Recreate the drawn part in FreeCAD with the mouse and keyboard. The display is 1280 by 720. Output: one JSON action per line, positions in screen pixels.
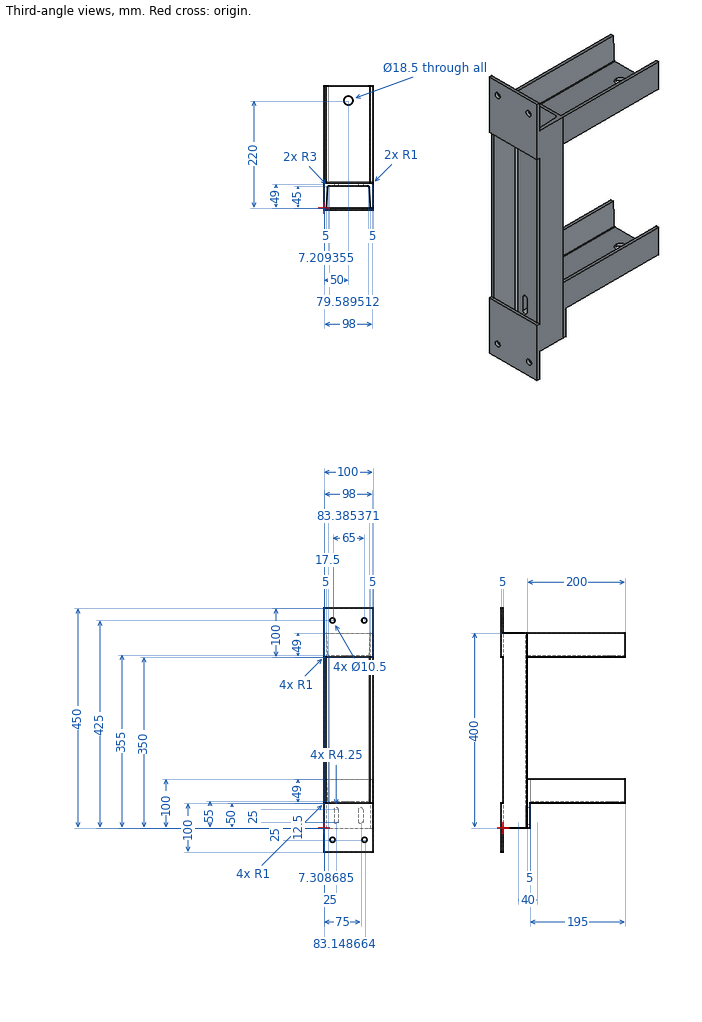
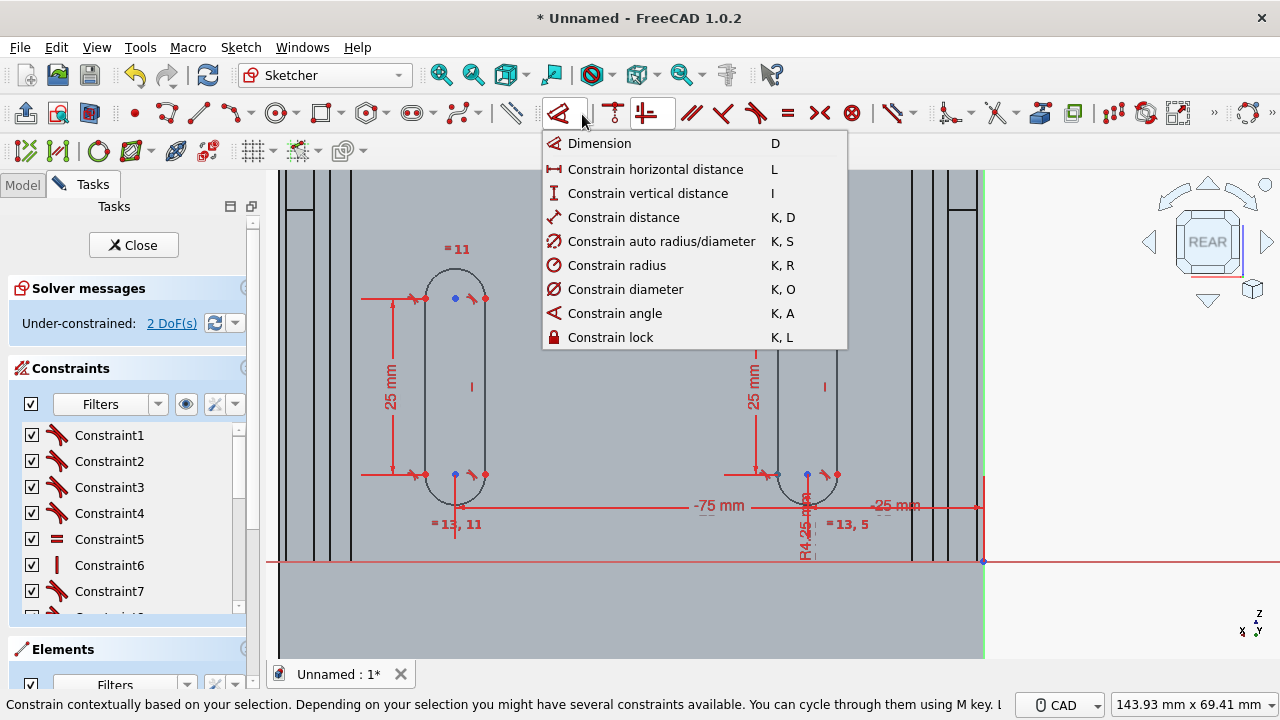
{"action": "left_click", "coordinate": [695, 193]}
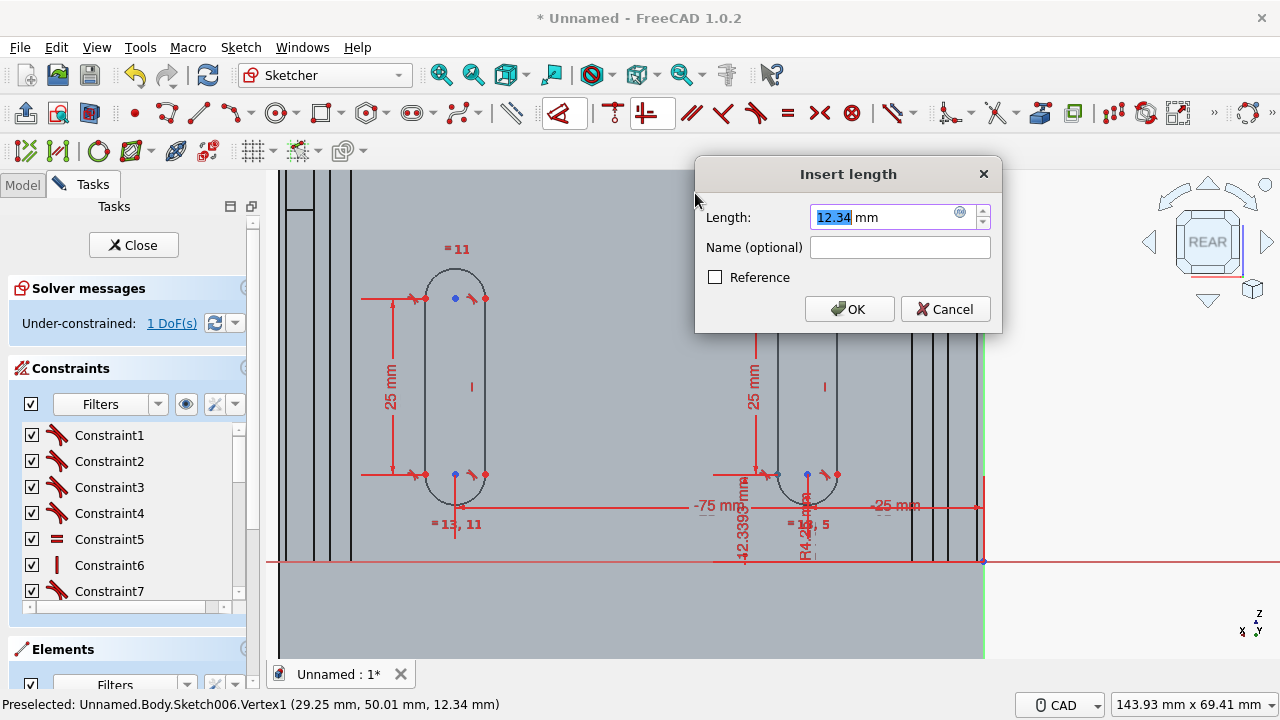
{"action": "type", "text": "12.5"}
{"action": "key", "text": "Return"}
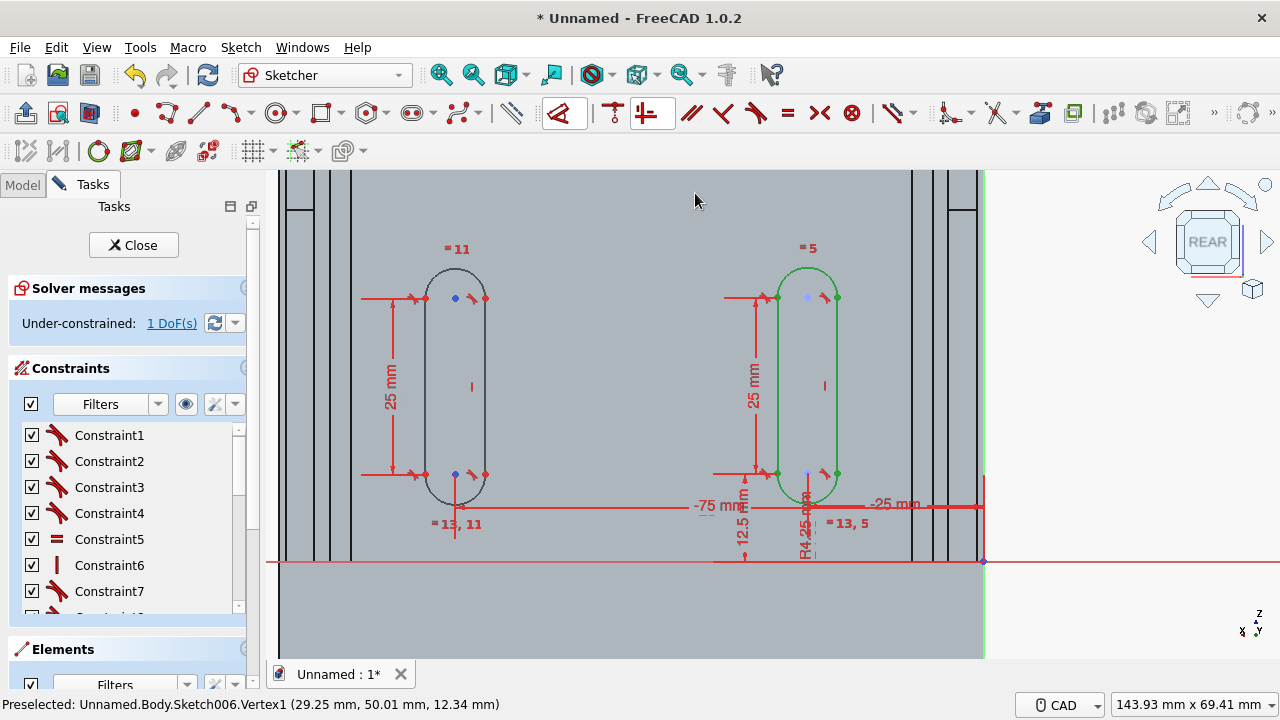
{"action": "left_click", "coordinate": [425, 475]}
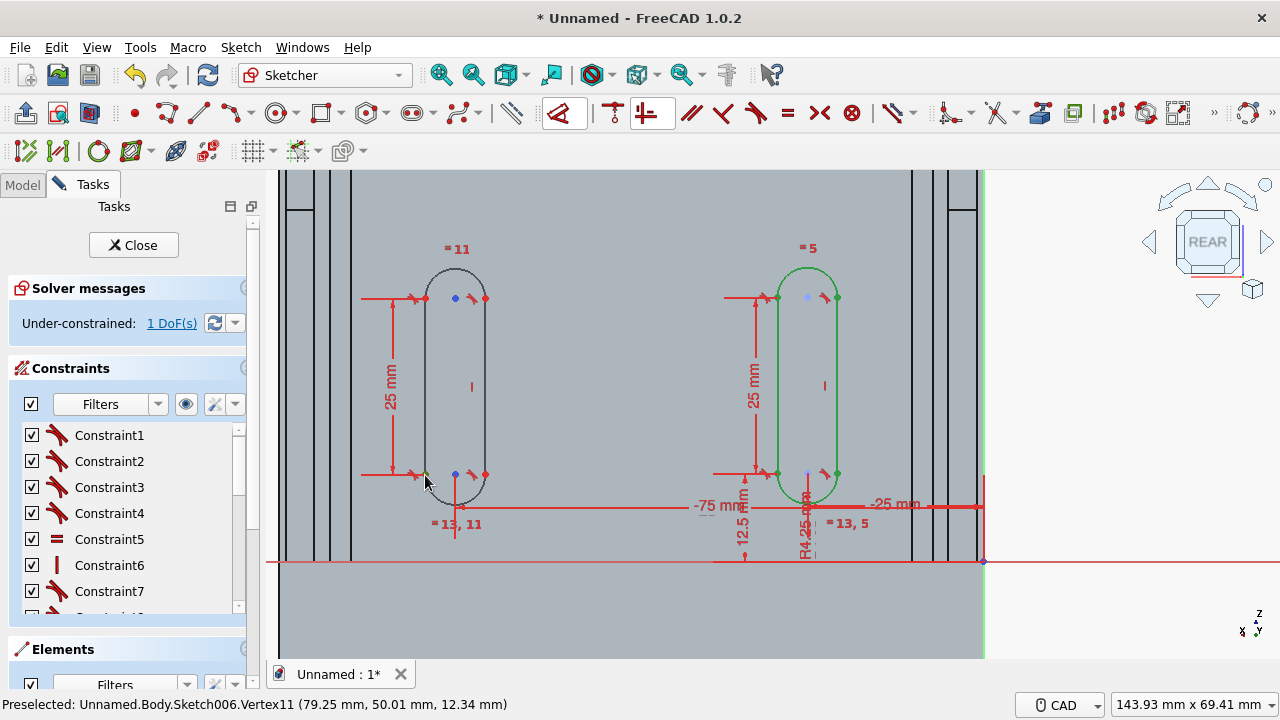
{"action": "key", "text": "i"}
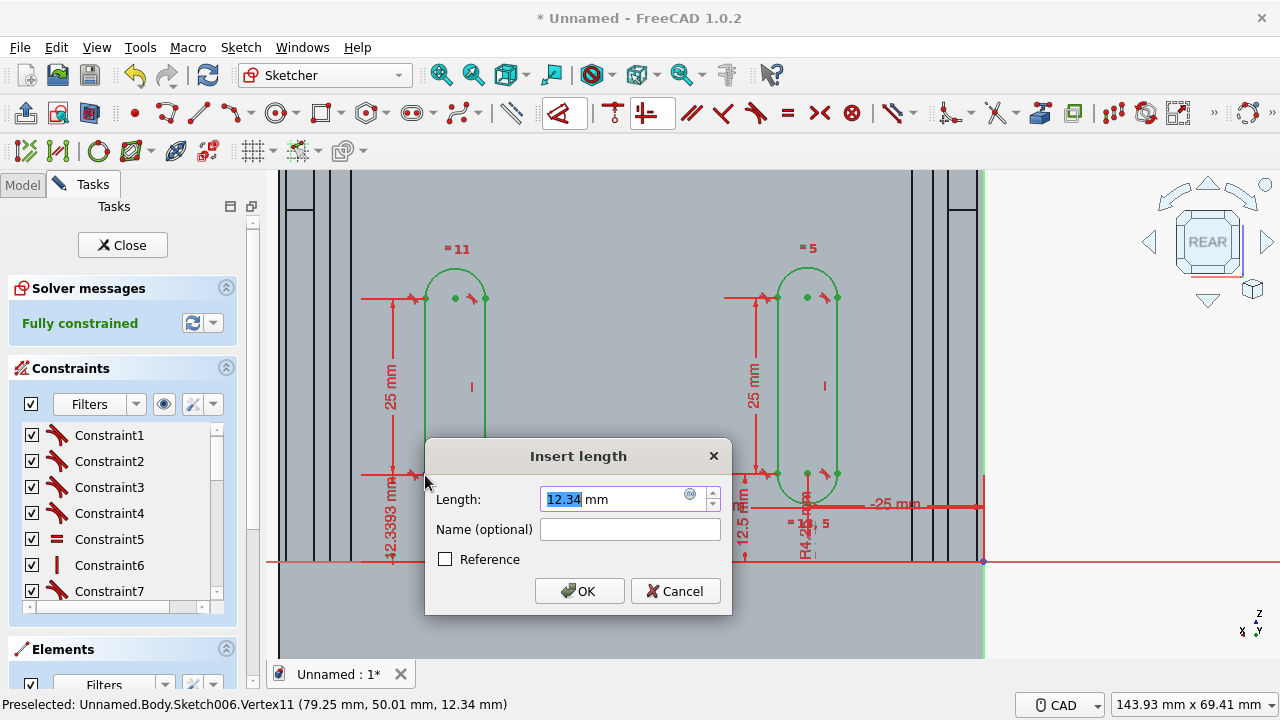
{"action": "type", "text": "12.5"}
{"action": "key", "text": "Return"}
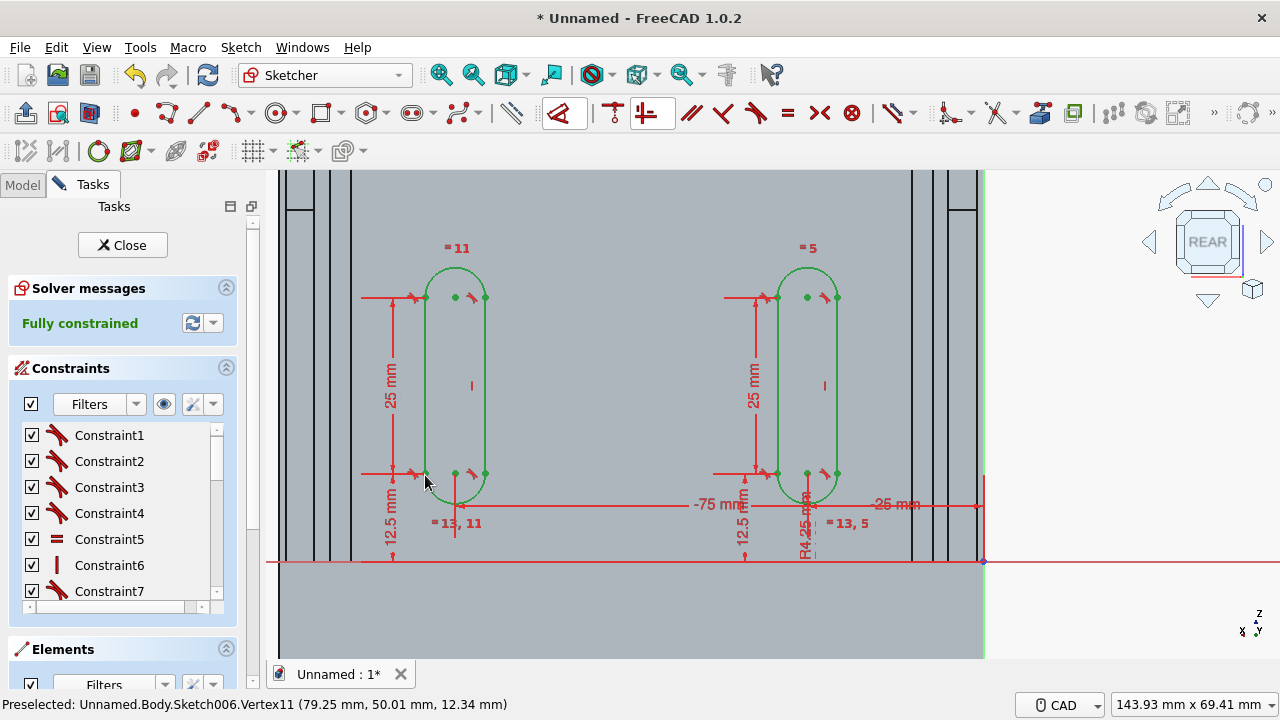
{"action": "left_click", "coordinate": [123, 245]}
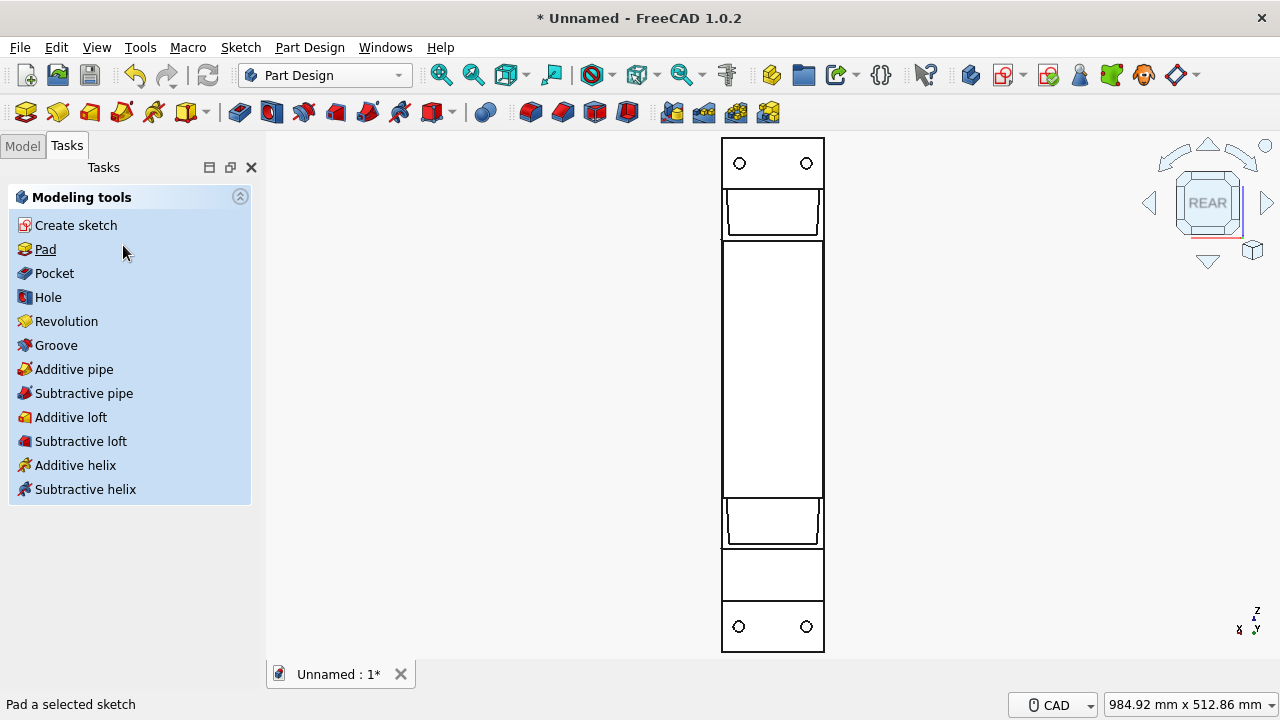
{"action": "left_click", "coordinate": [240, 112]}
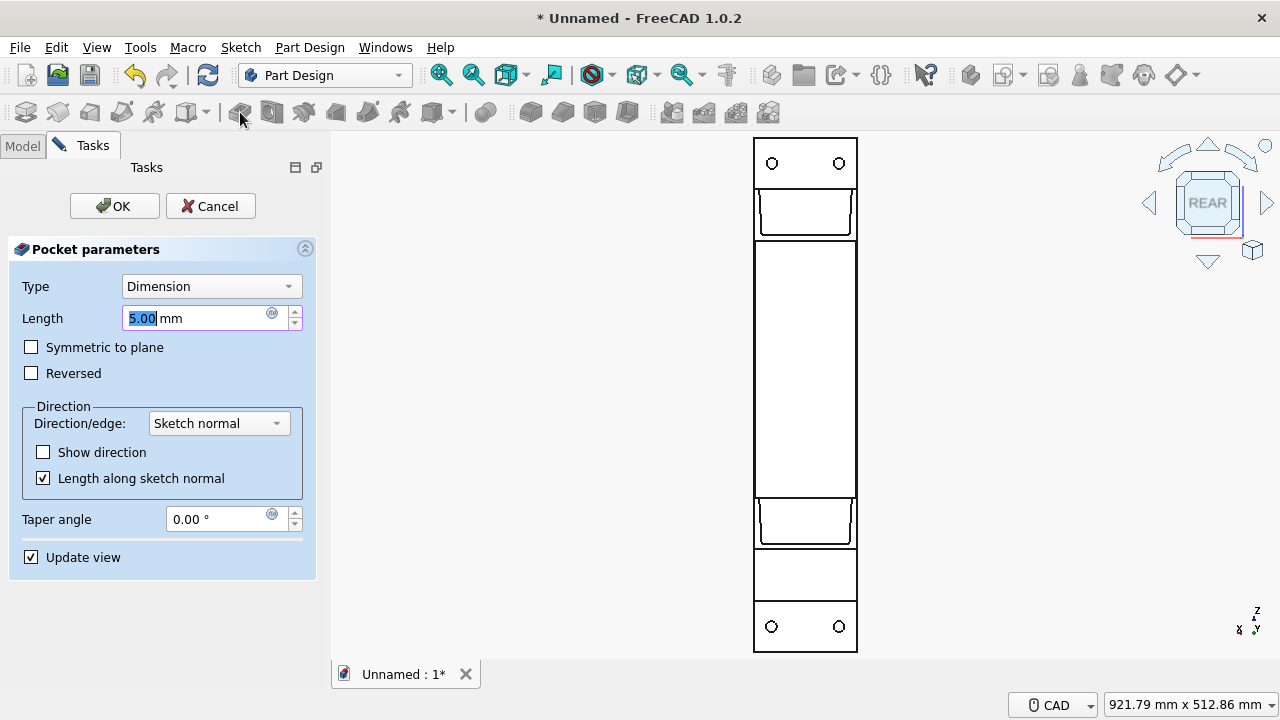
{"action": "type", "text": "40"}
{"action": "key", "text": "Tab"}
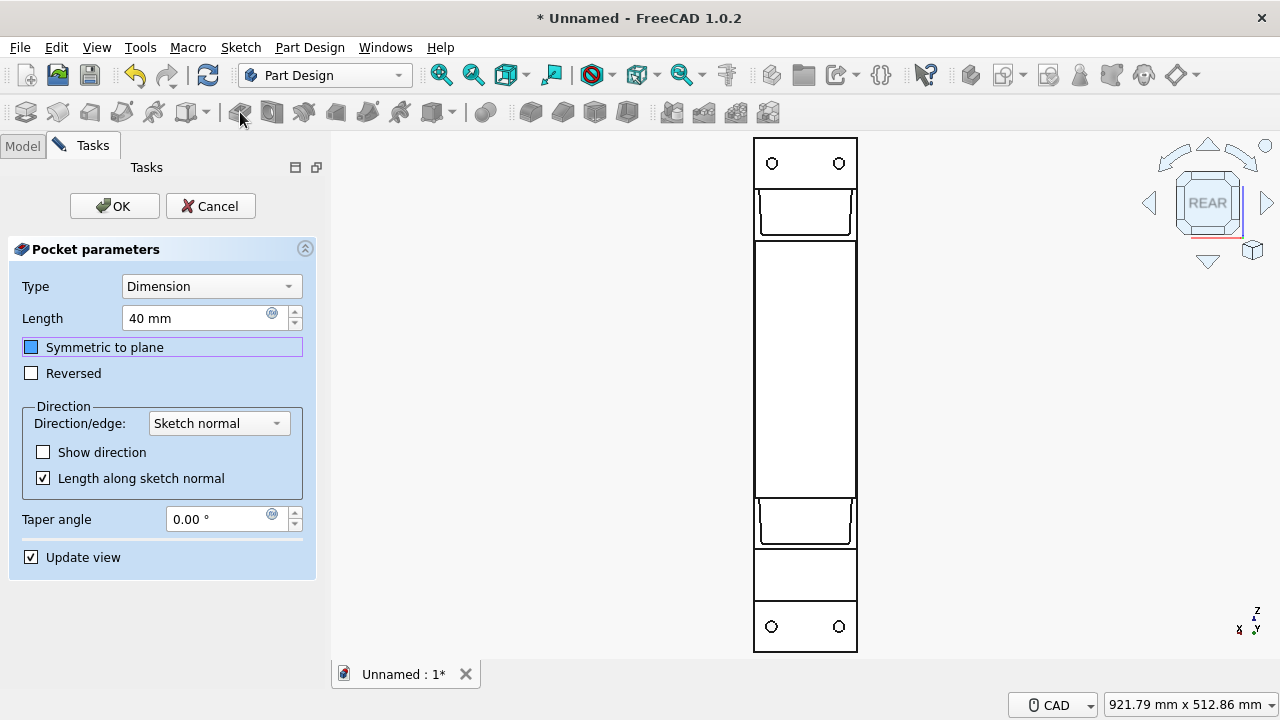
{"action": "left_click", "coordinate": [30, 347]}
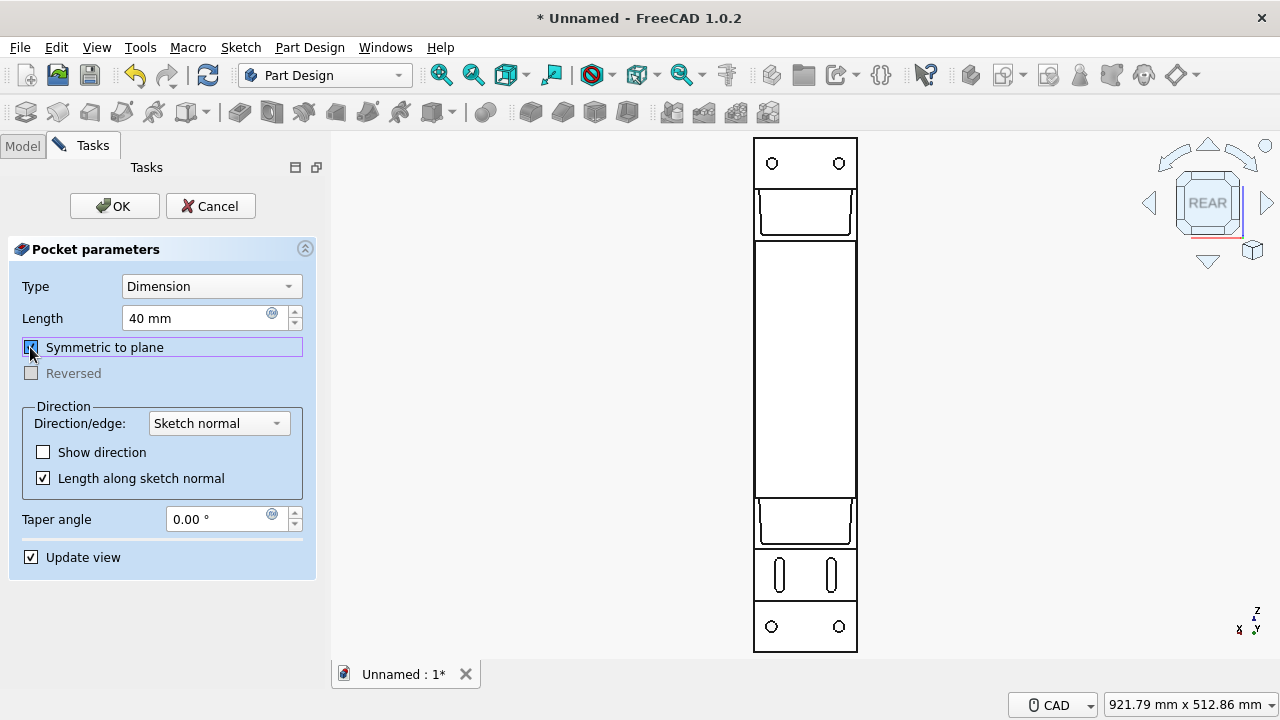
{"action": "left_click", "coordinate": [115, 206]}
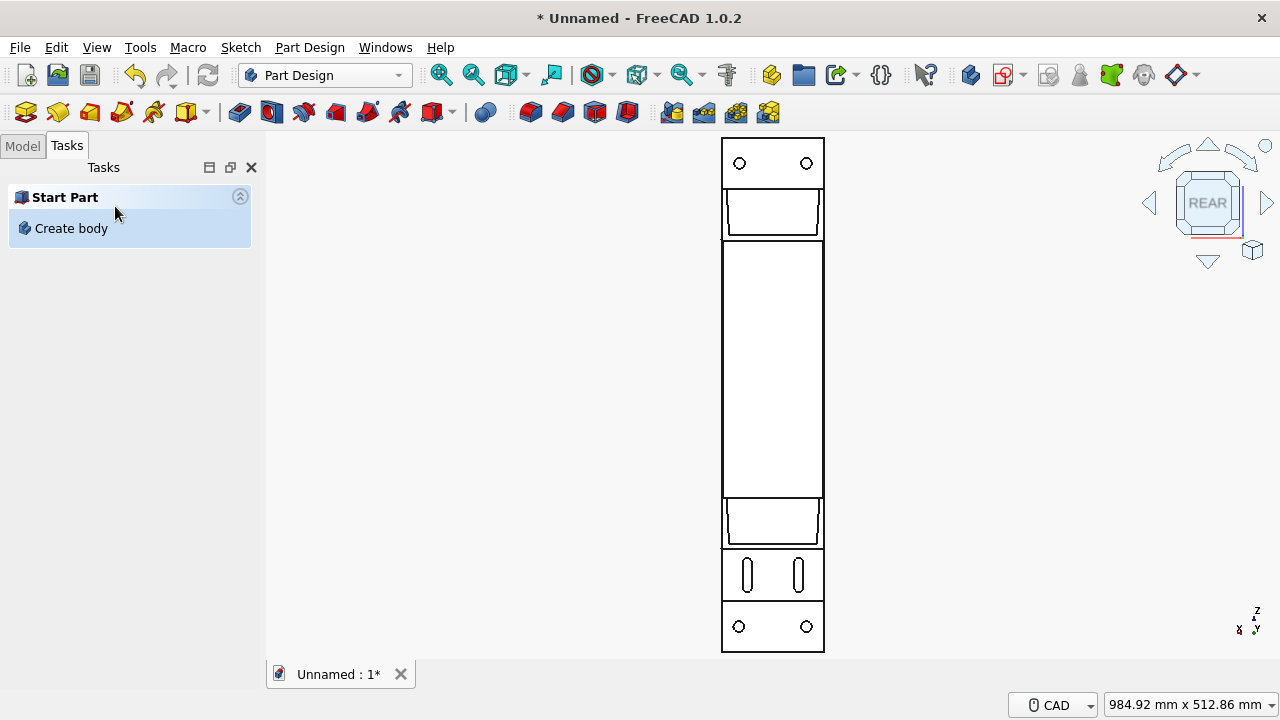
{"action": "key", "text": "5"}